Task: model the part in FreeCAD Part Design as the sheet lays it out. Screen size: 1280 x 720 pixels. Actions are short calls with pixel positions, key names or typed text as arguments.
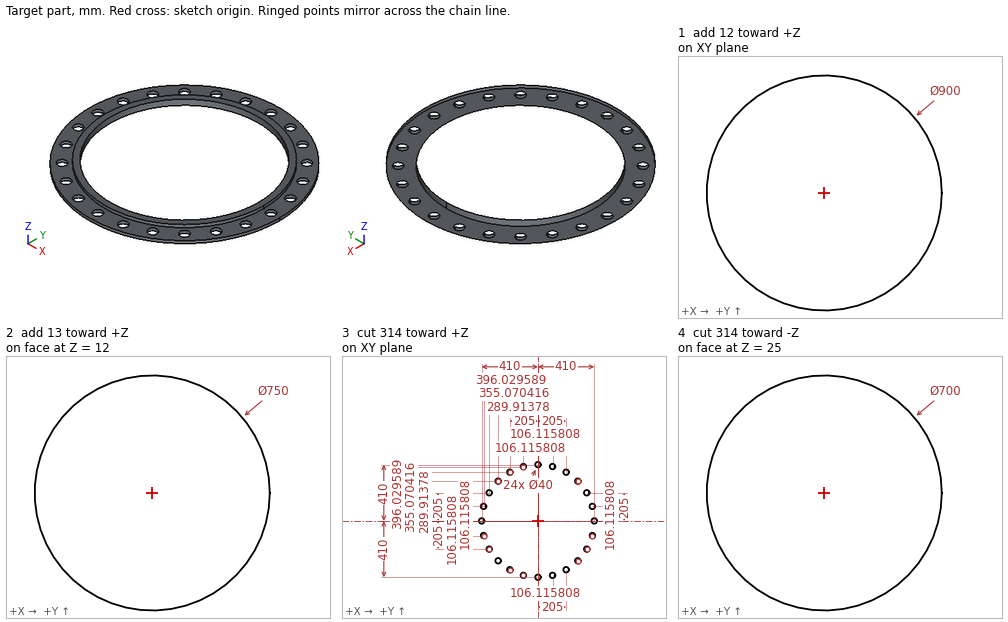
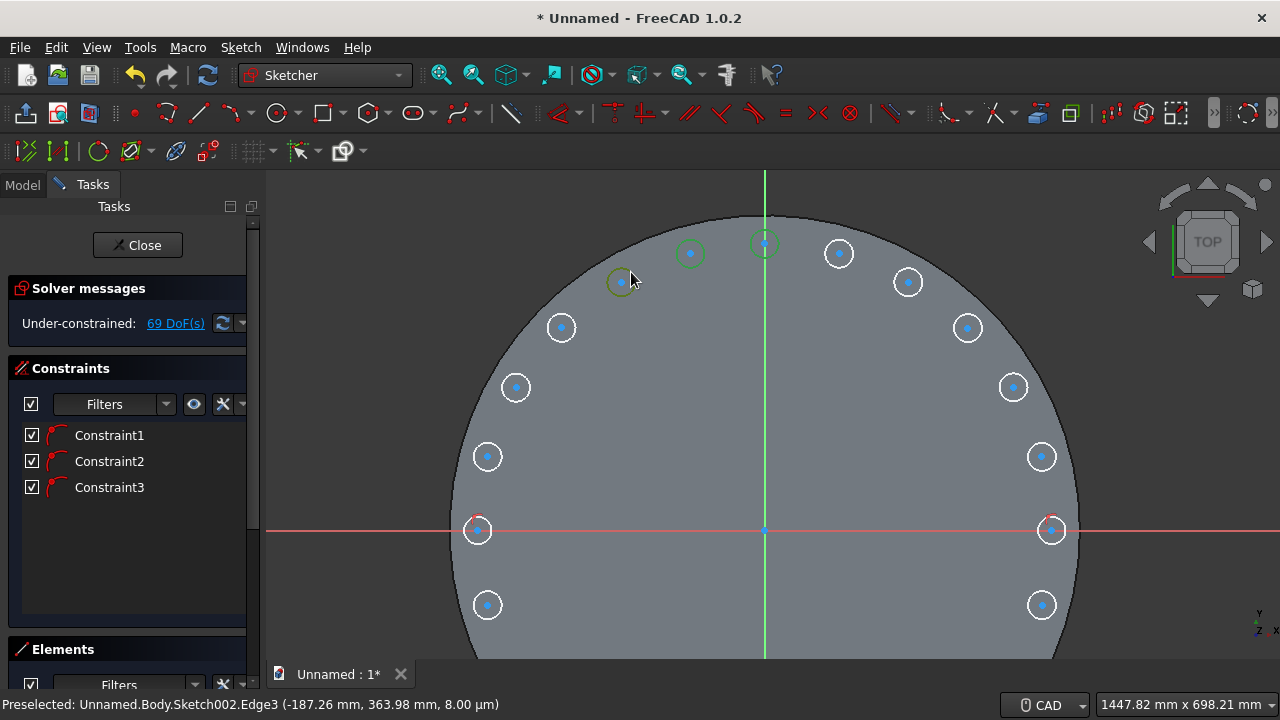
click(571, 318)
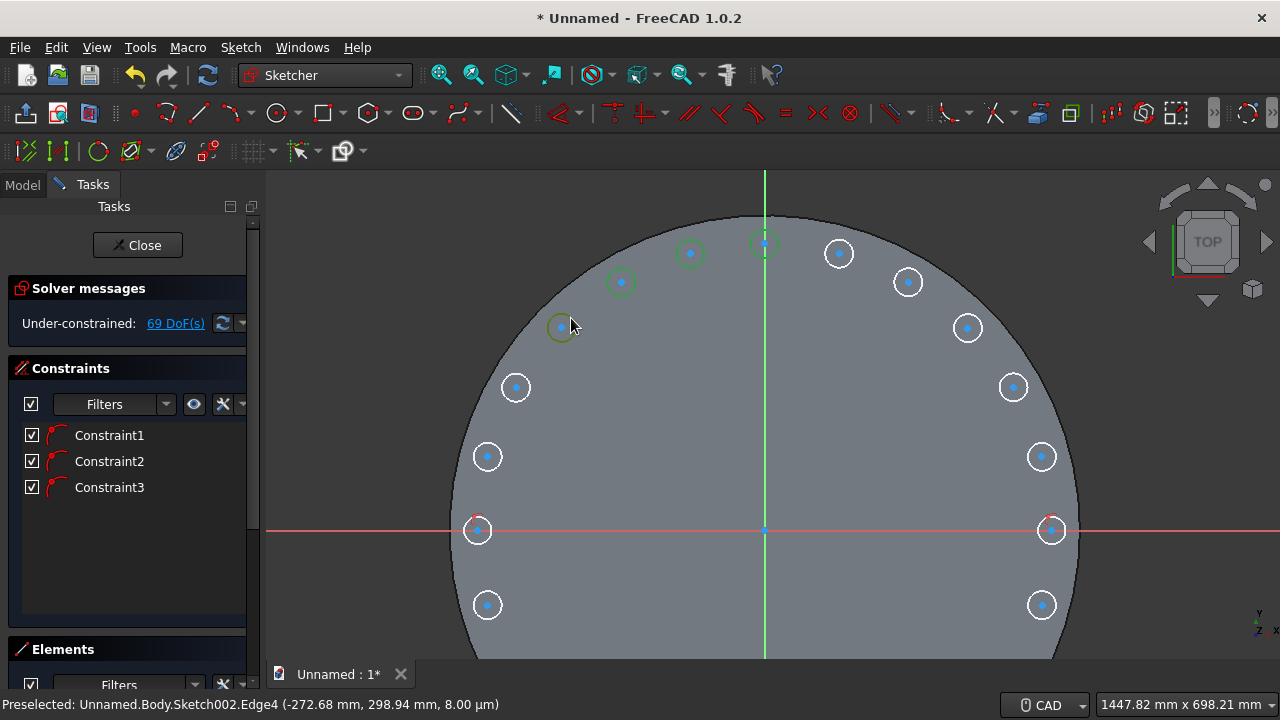
click(526, 378)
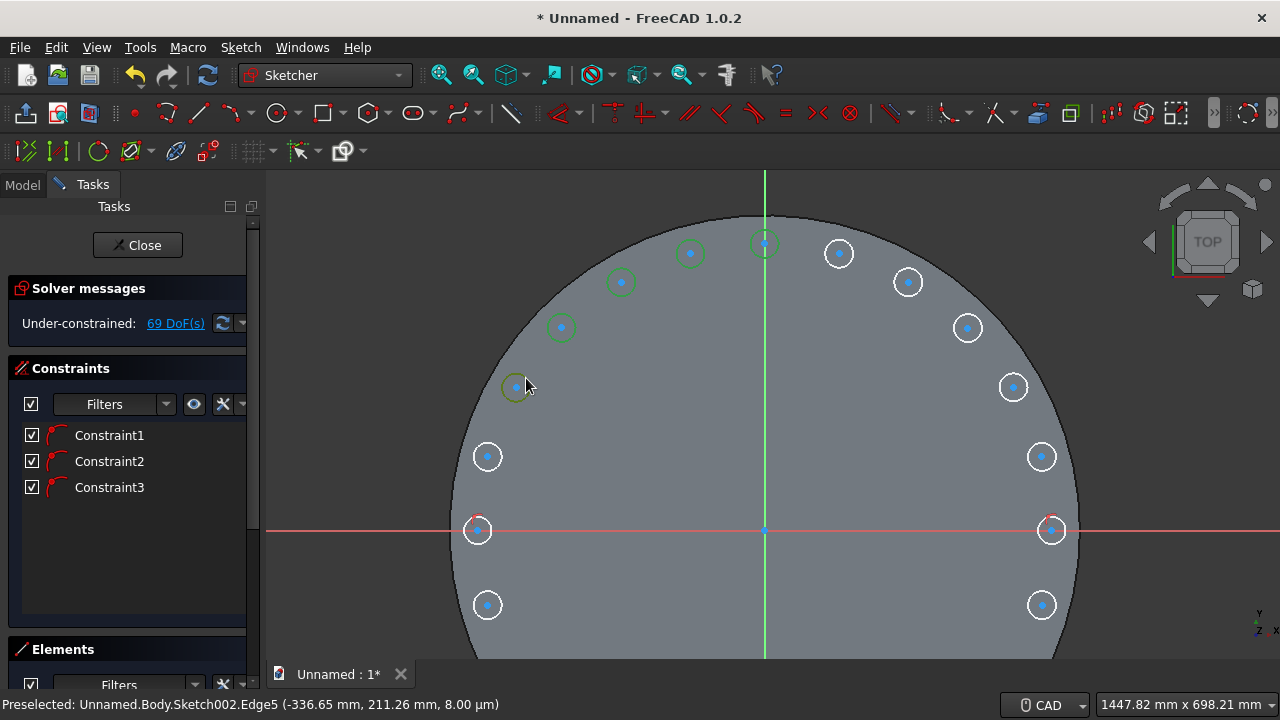
click(498, 447)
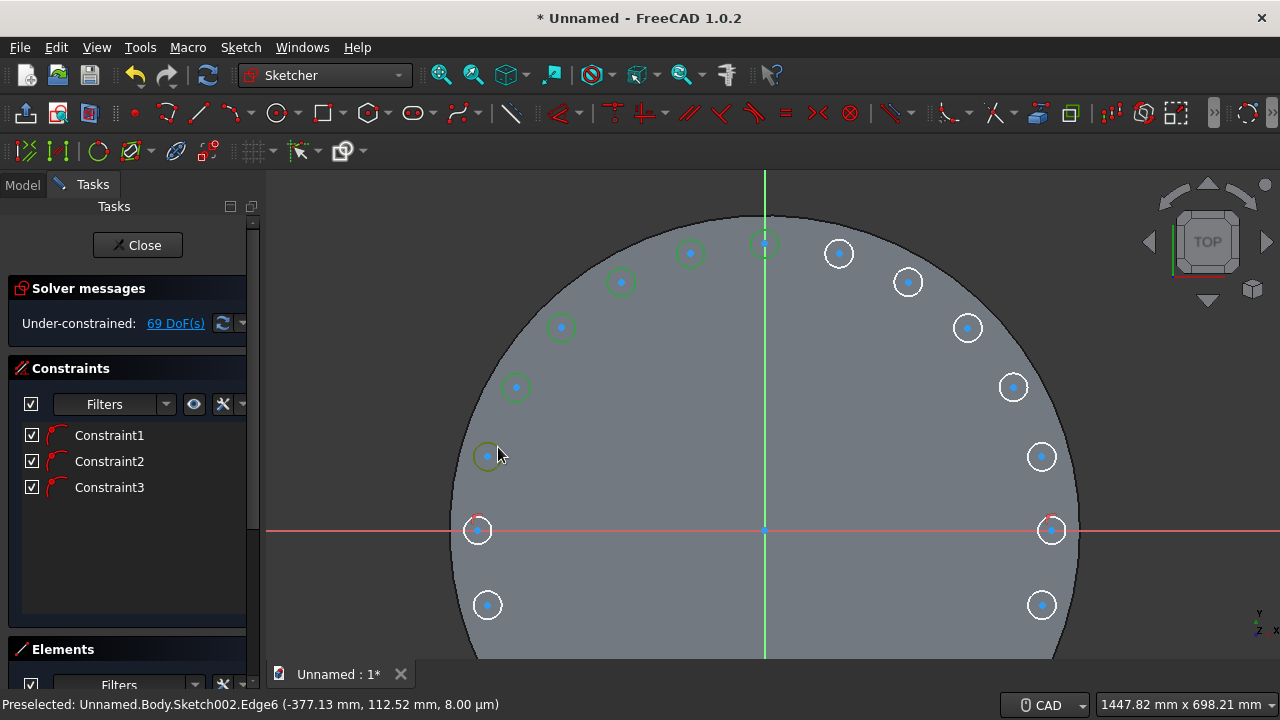
scroll(487, 521, up, 2)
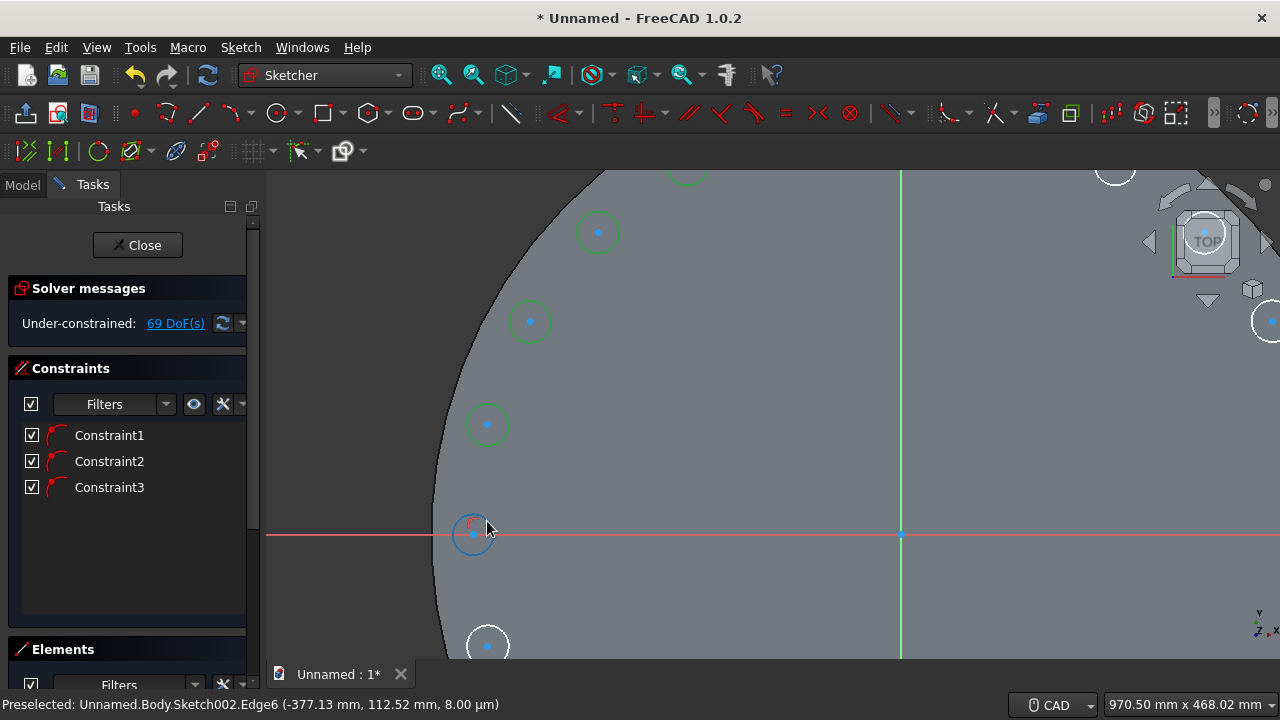
click(488, 520)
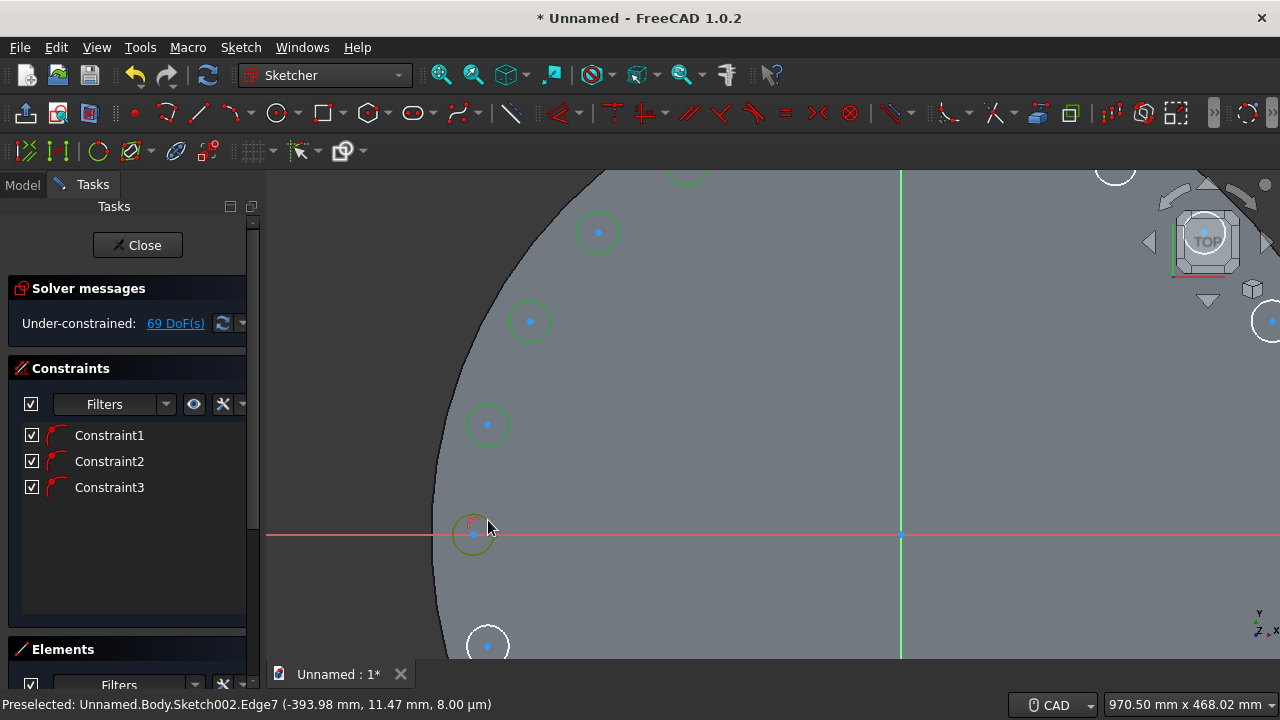
click(488, 625)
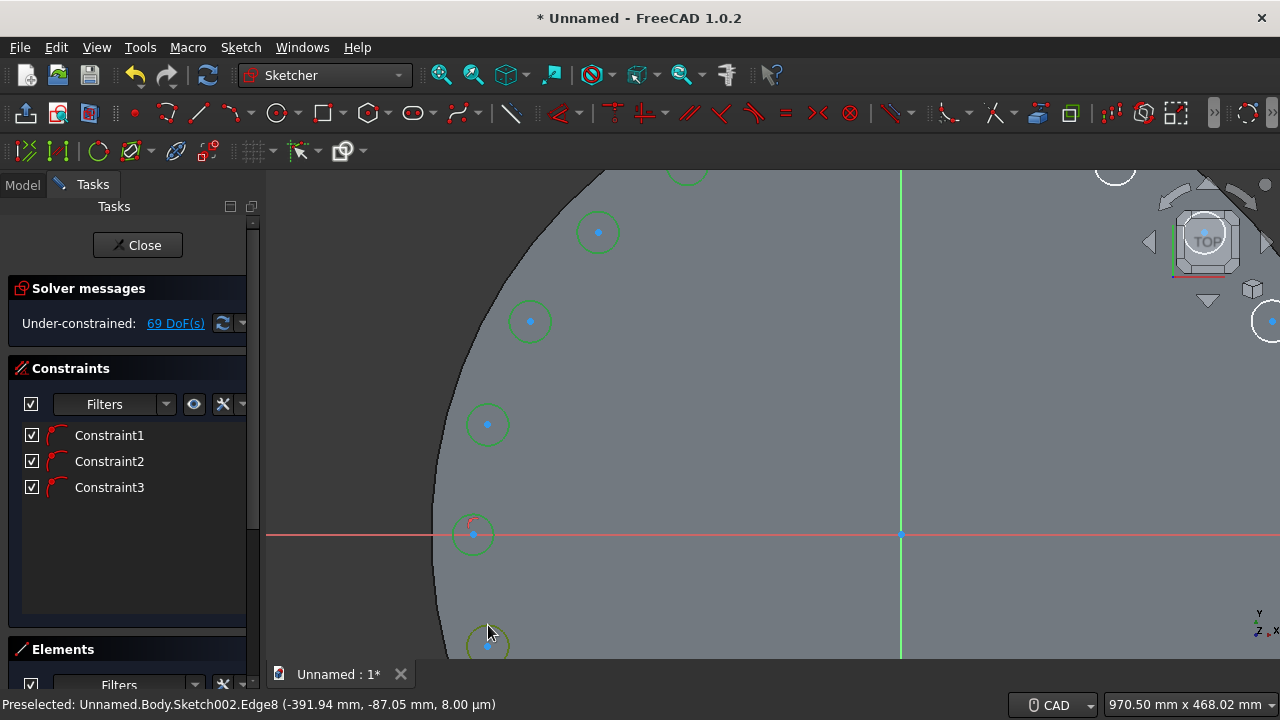
scroll(590, 344, down, 5)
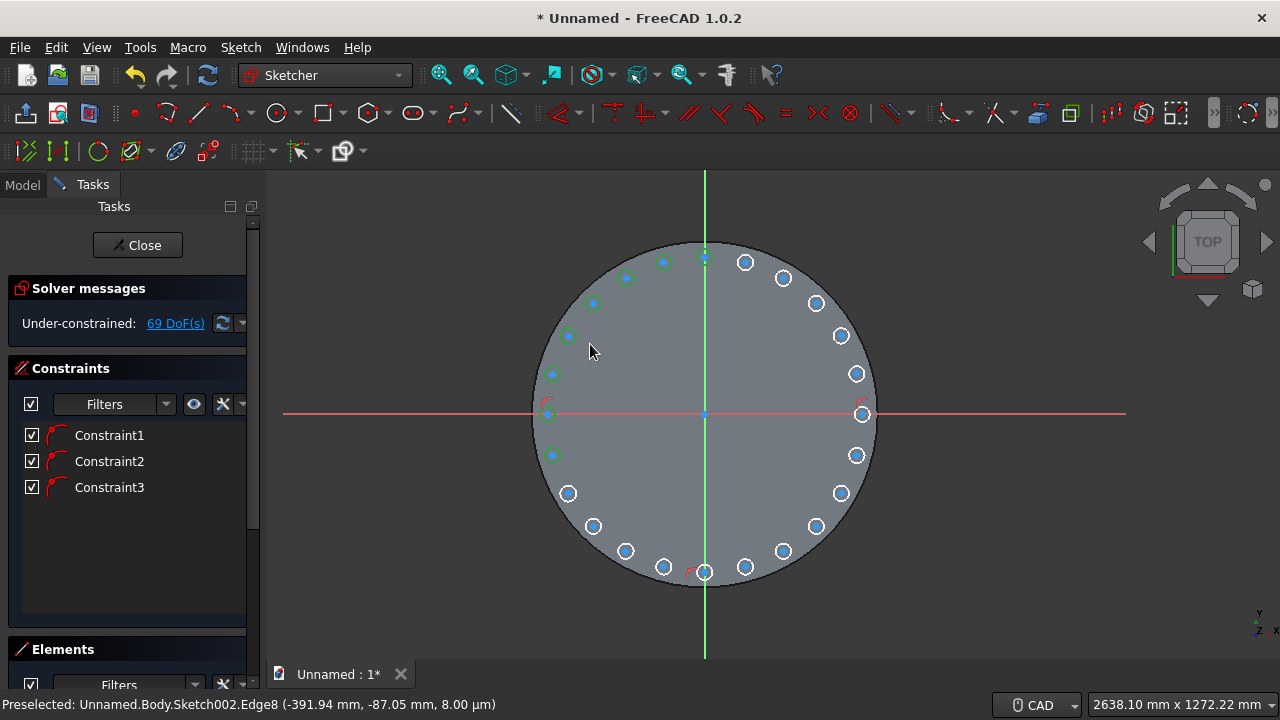
scroll(574, 488, up, 3)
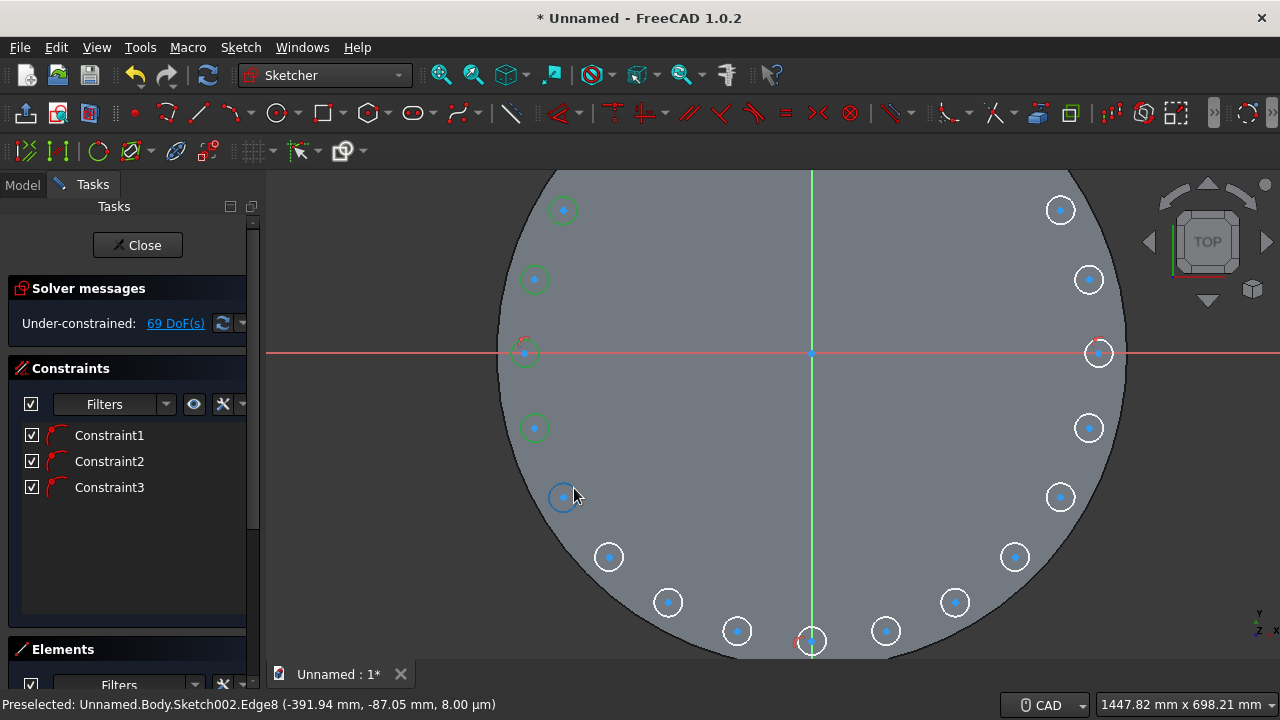
click(573, 488)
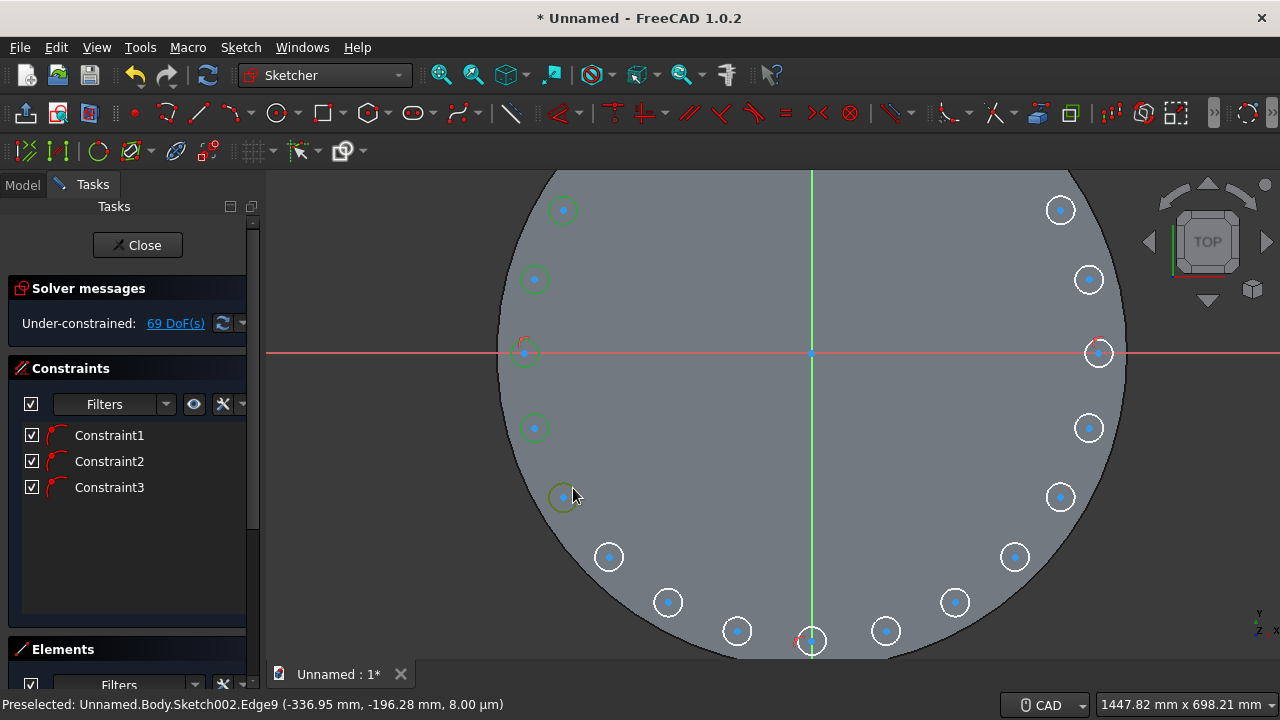
click(619, 547)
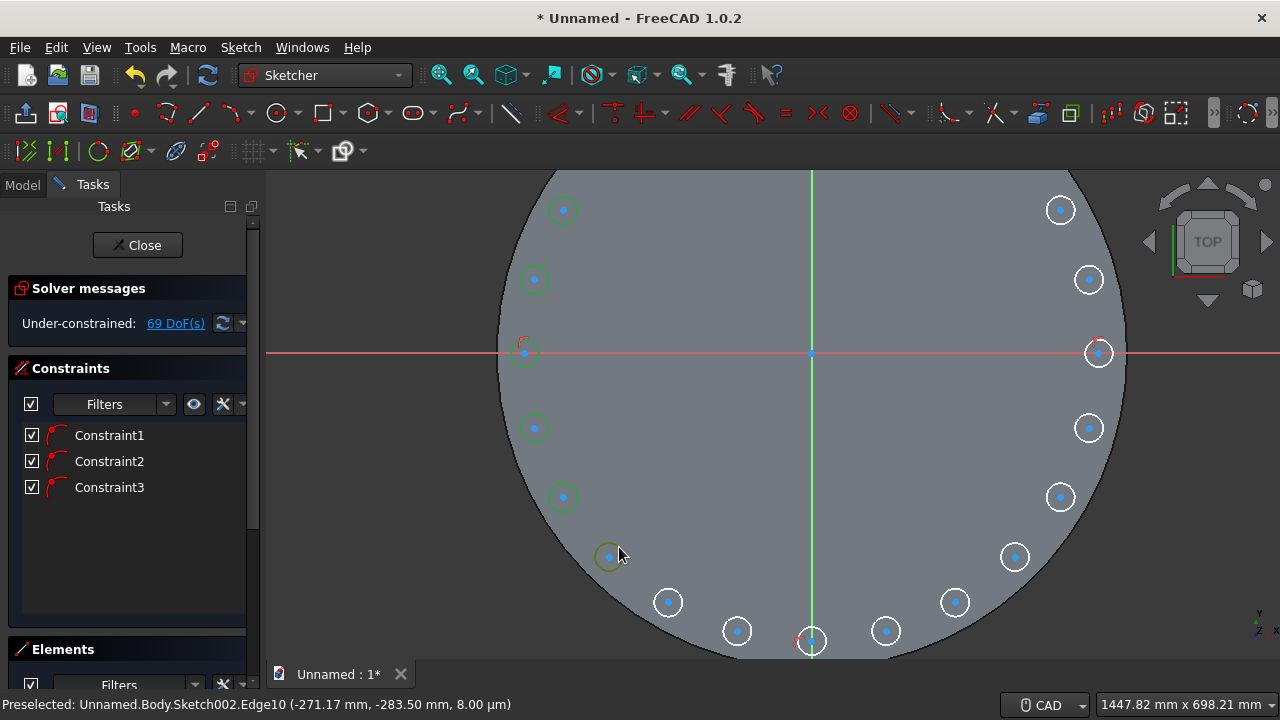
click(678, 593)